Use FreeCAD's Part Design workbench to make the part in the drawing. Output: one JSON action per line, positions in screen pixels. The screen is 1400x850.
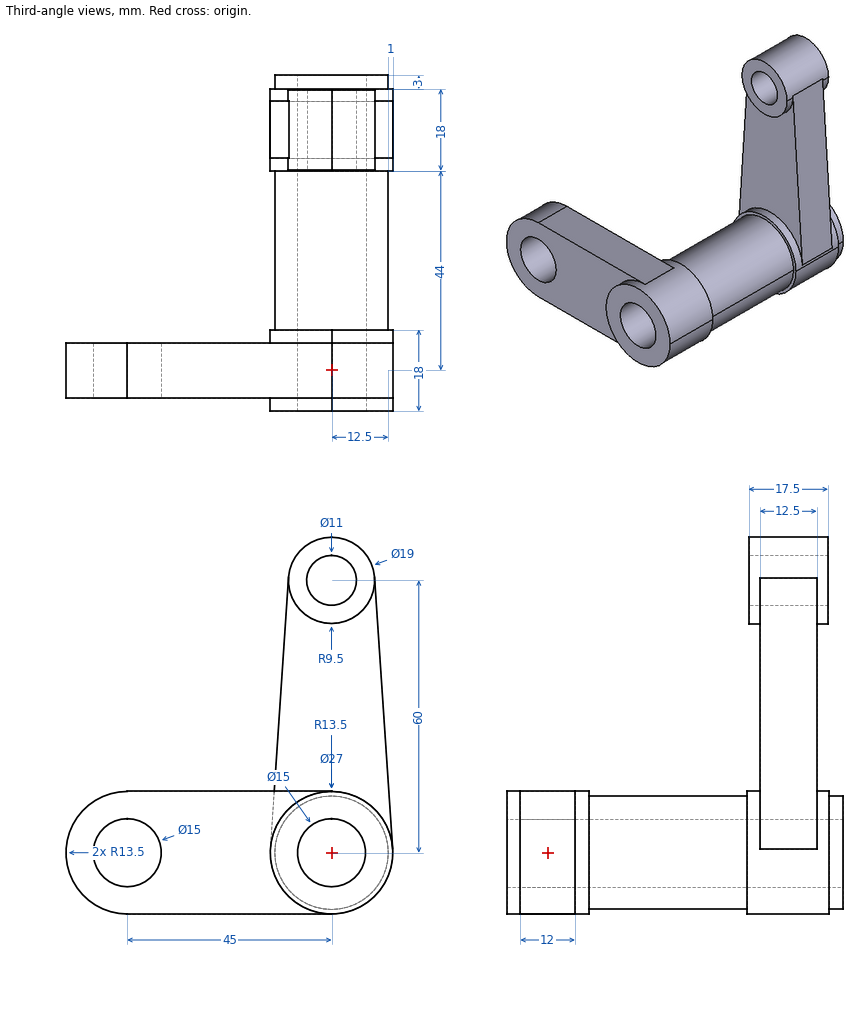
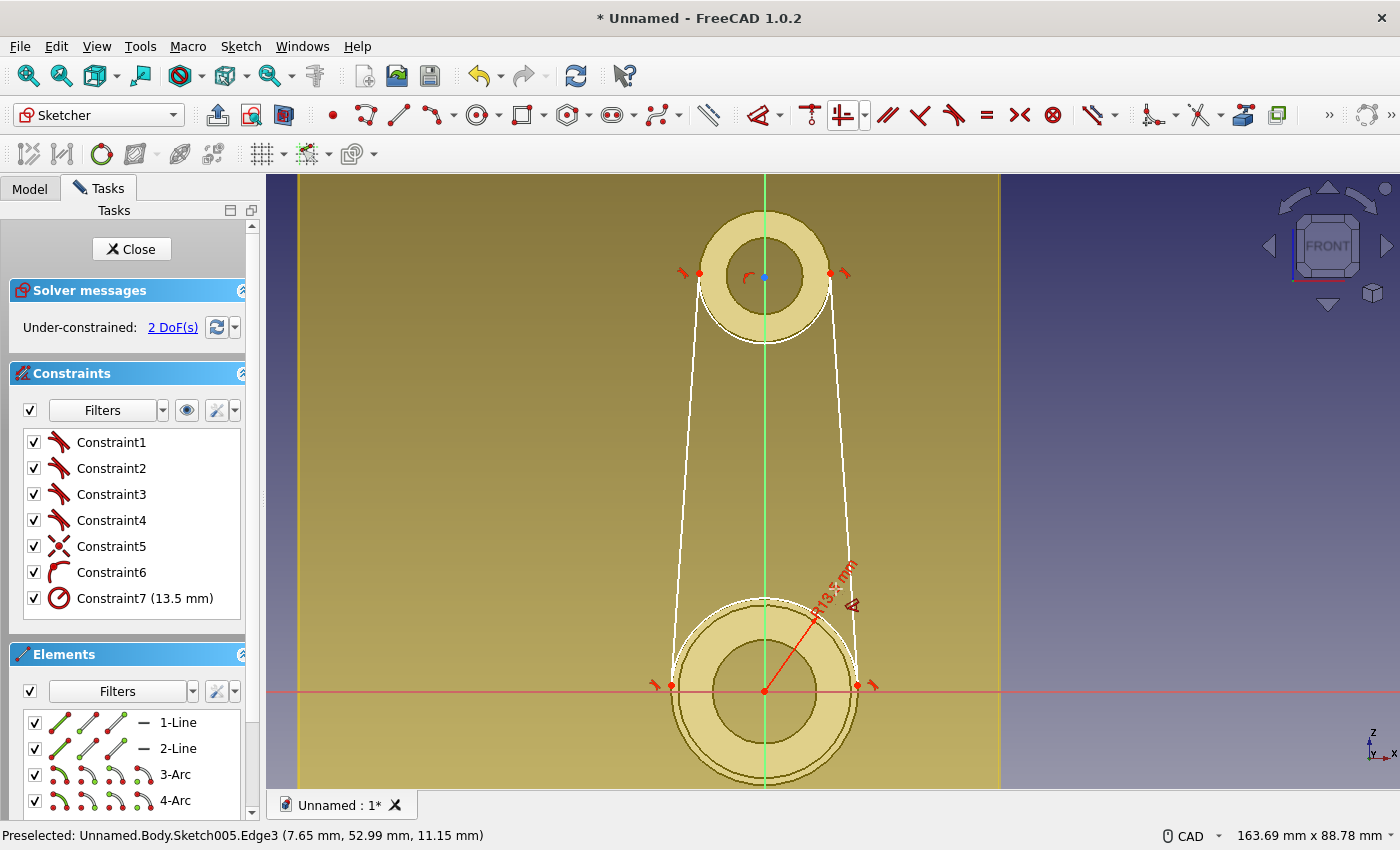
{"action": "left_click", "coordinate": [725, 330]}
{"action": "left_click", "coordinate": [676, 318]}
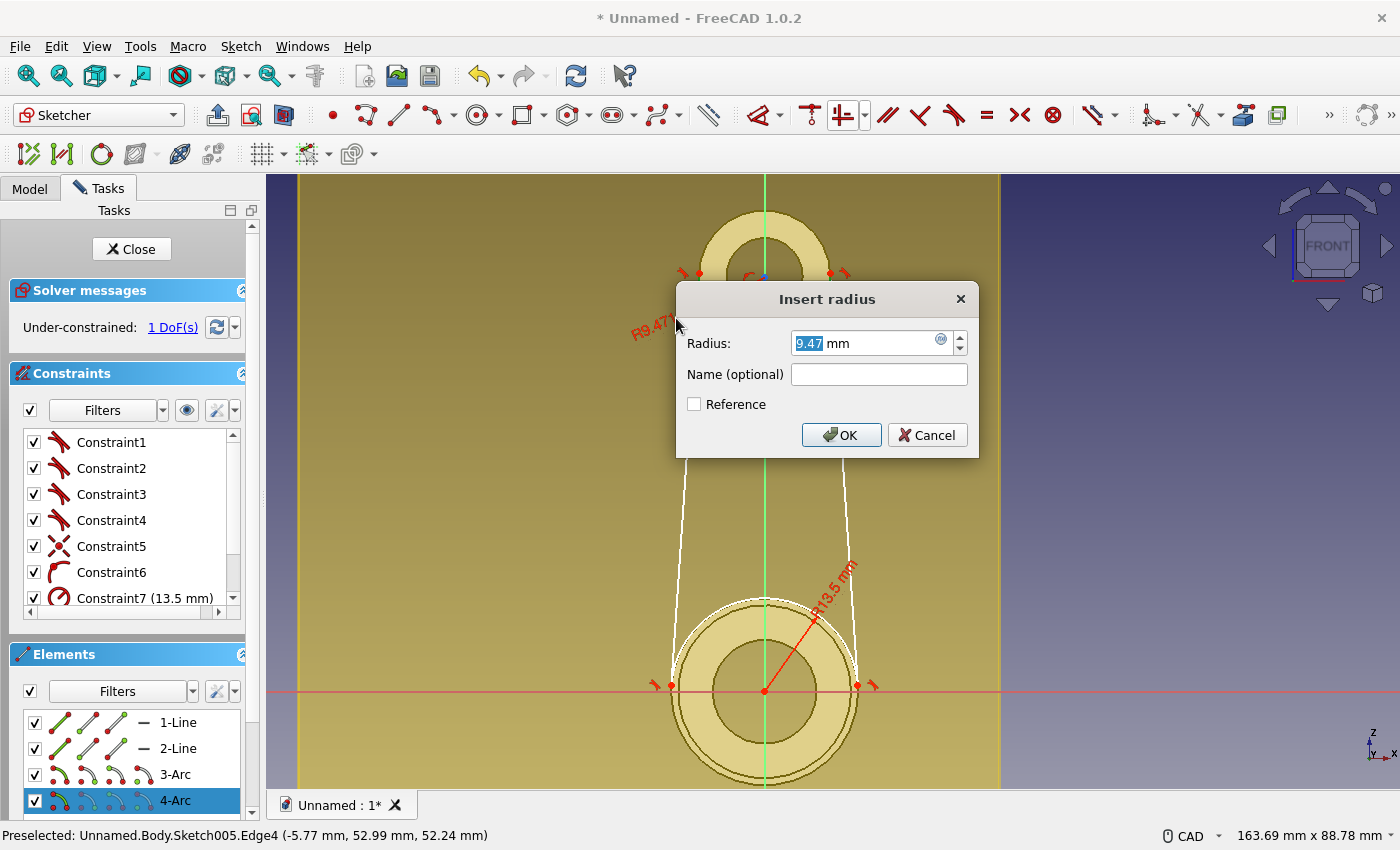
{"action": "type", "text": "9.5"}
{"action": "key", "text": "Return"}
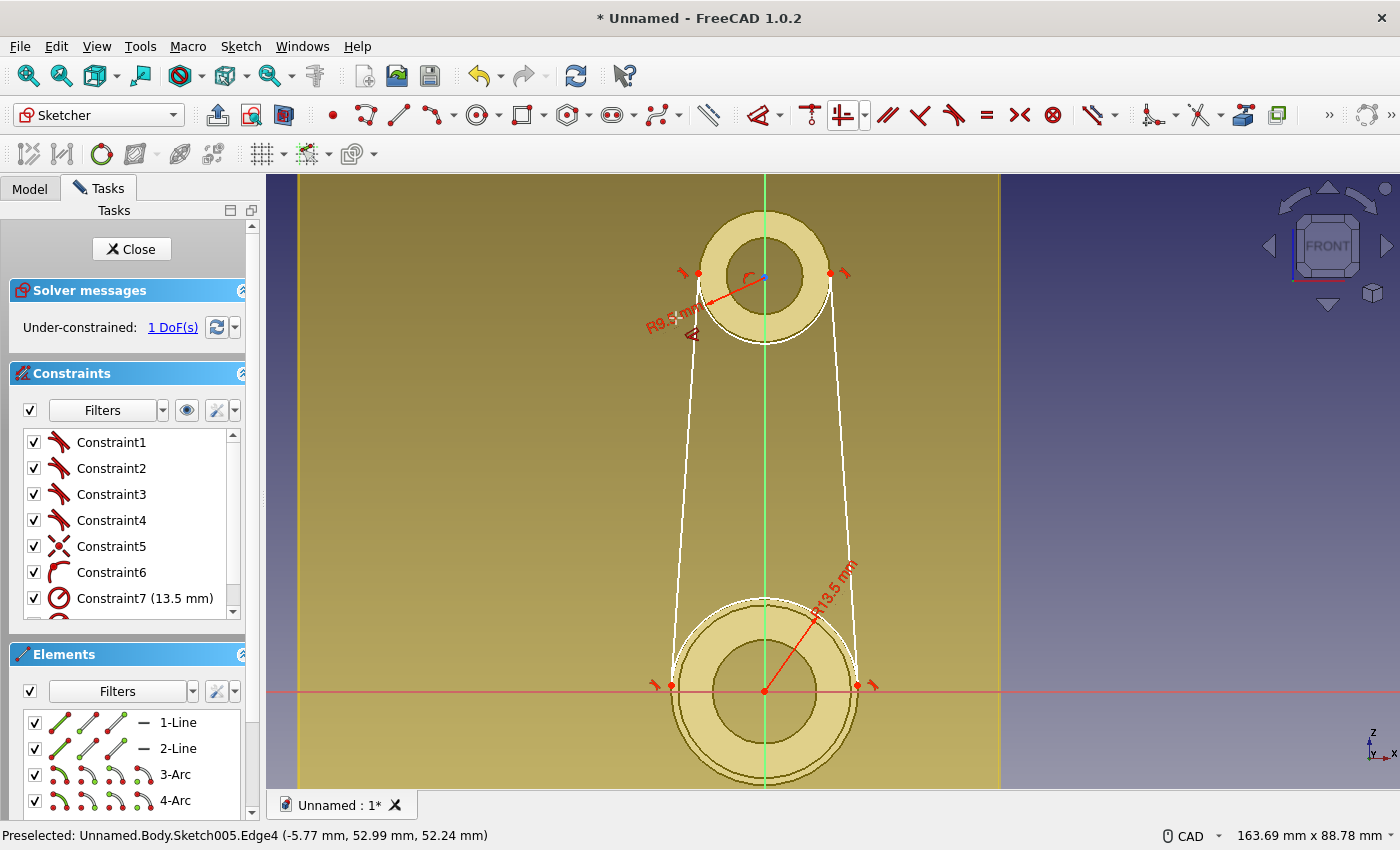
{"action": "left_click", "coordinate": [765, 278]}
{"action": "left_click", "coordinate": [799, 485]}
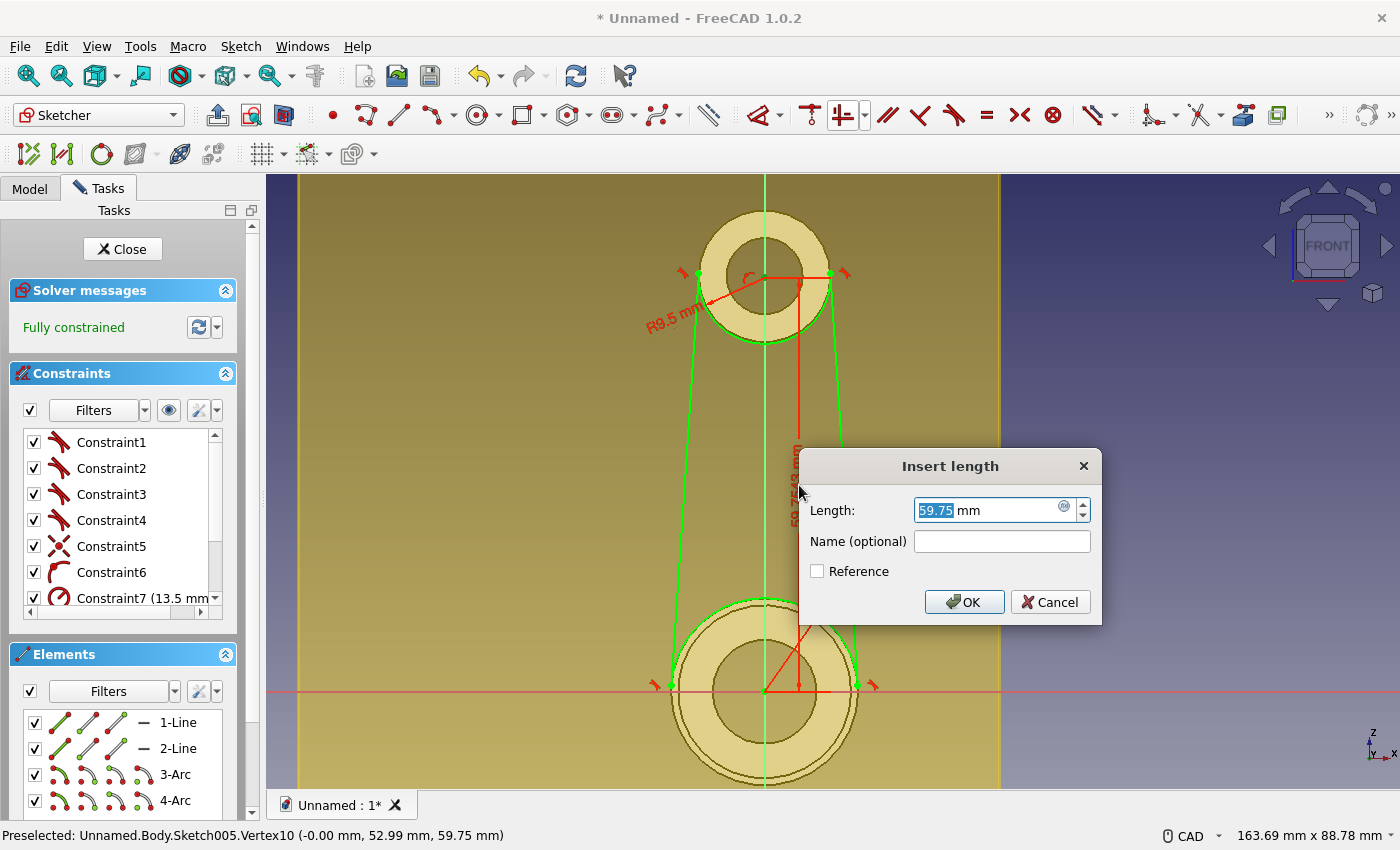
{"action": "type", "text": "60"}
{"action": "key", "text": "Return"}
{"action": "key", "text": "Escape"}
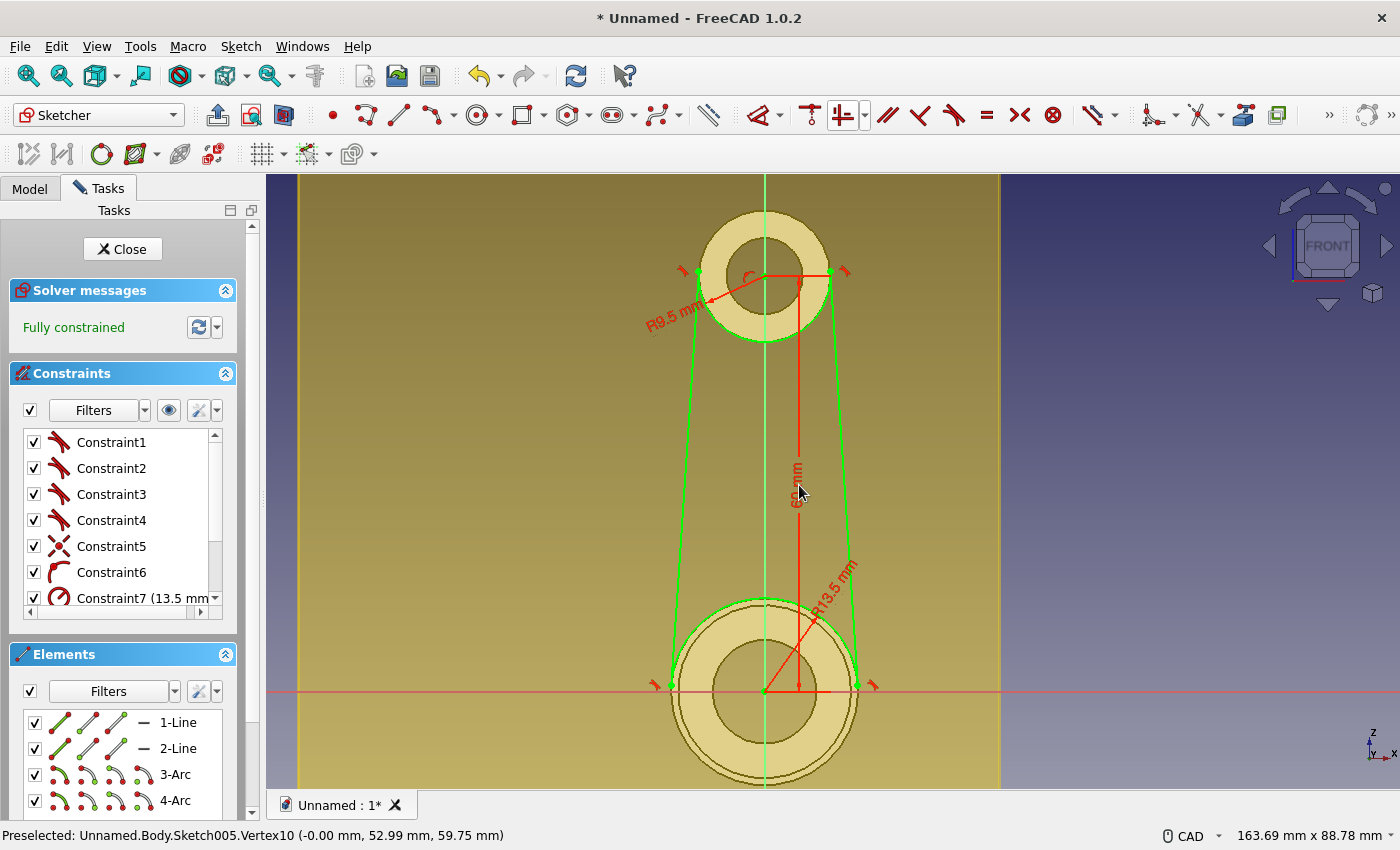
{"action": "left_click", "coordinate": [123, 249]}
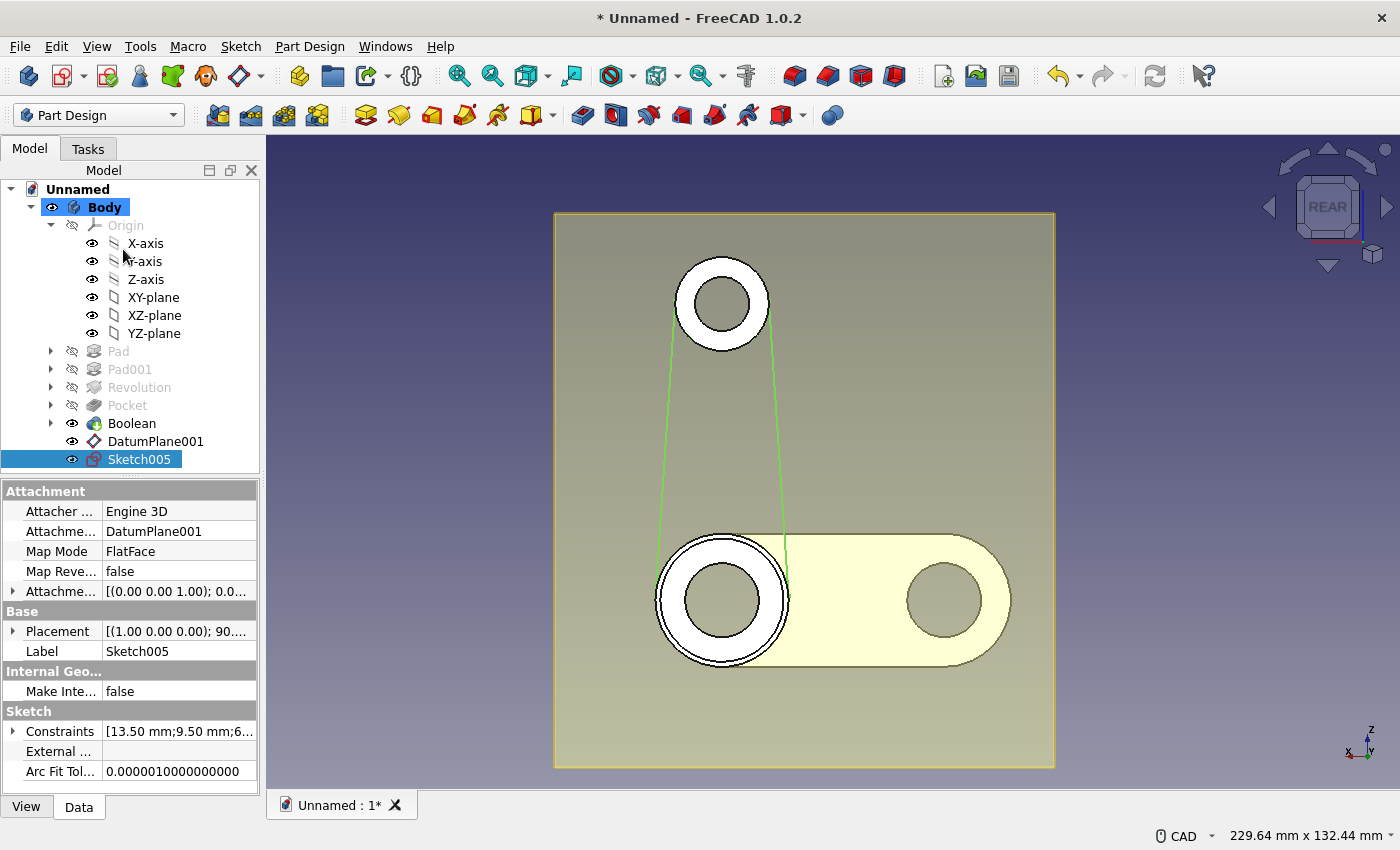
{"action": "left_click", "coordinate": [366, 116]}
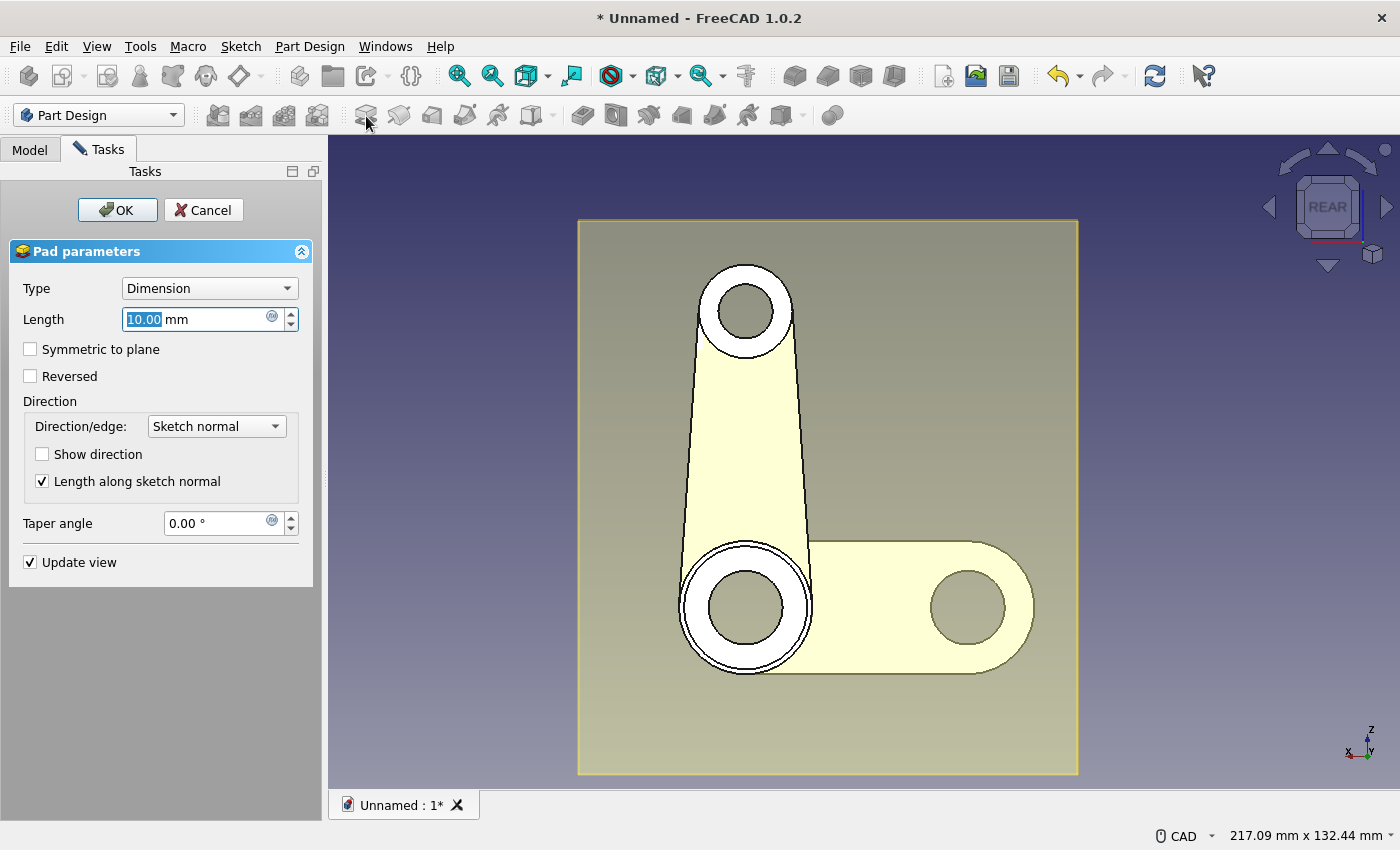
{"action": "type", "text": "12.5"}
{"action": "key", "text": "Tab"}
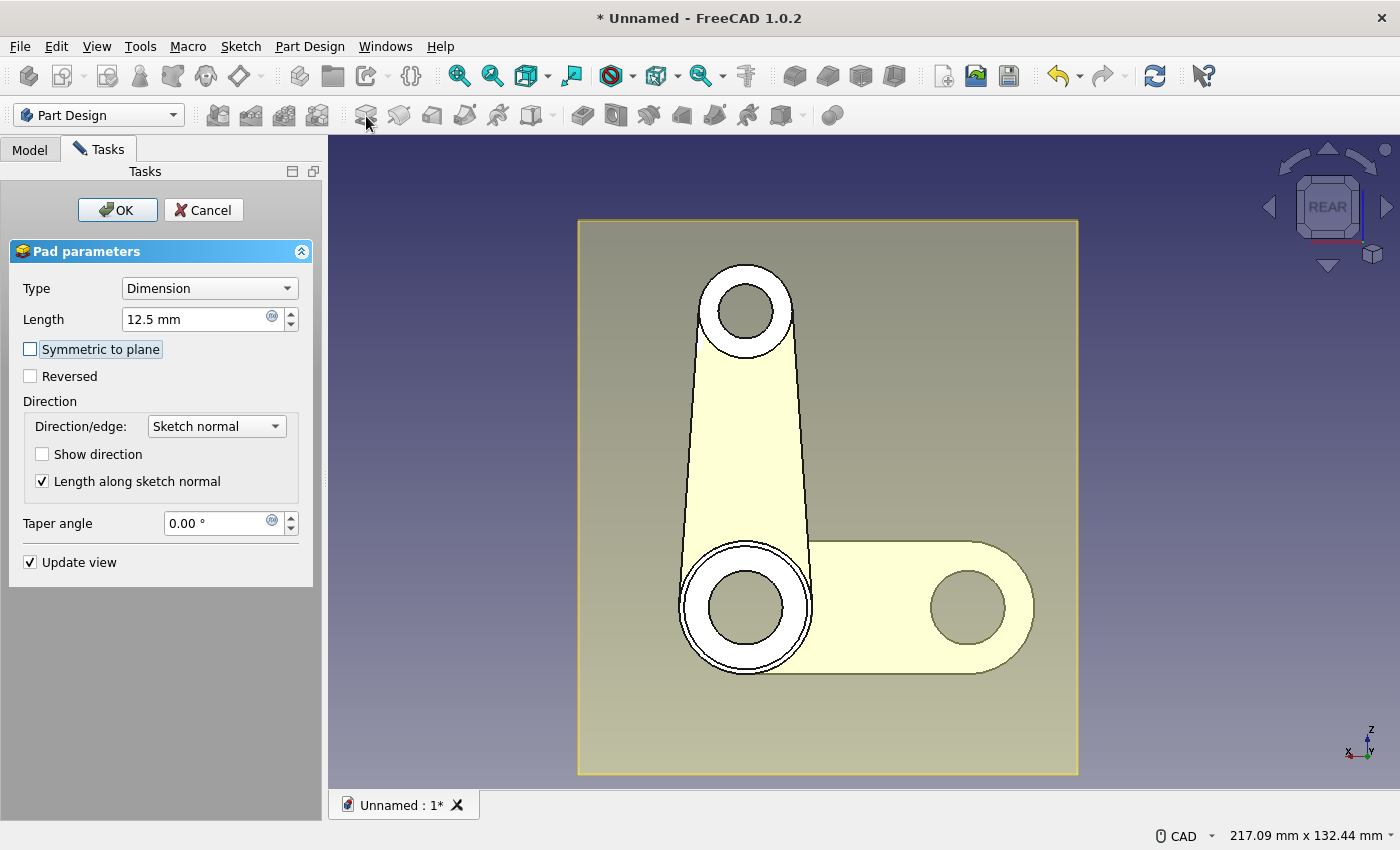
{"action": "left_click", "coordinate": [31, 349]}